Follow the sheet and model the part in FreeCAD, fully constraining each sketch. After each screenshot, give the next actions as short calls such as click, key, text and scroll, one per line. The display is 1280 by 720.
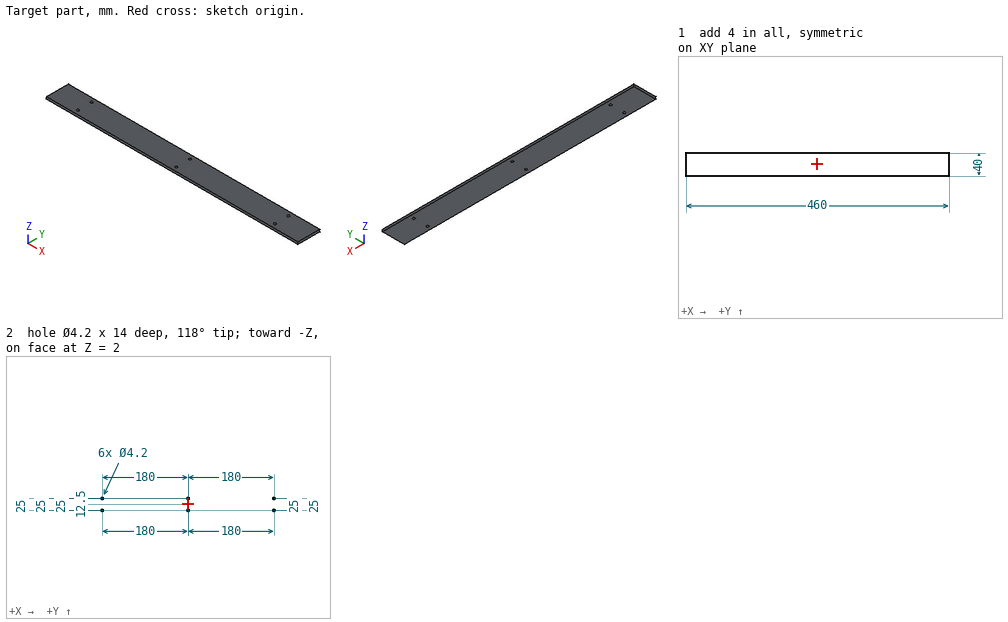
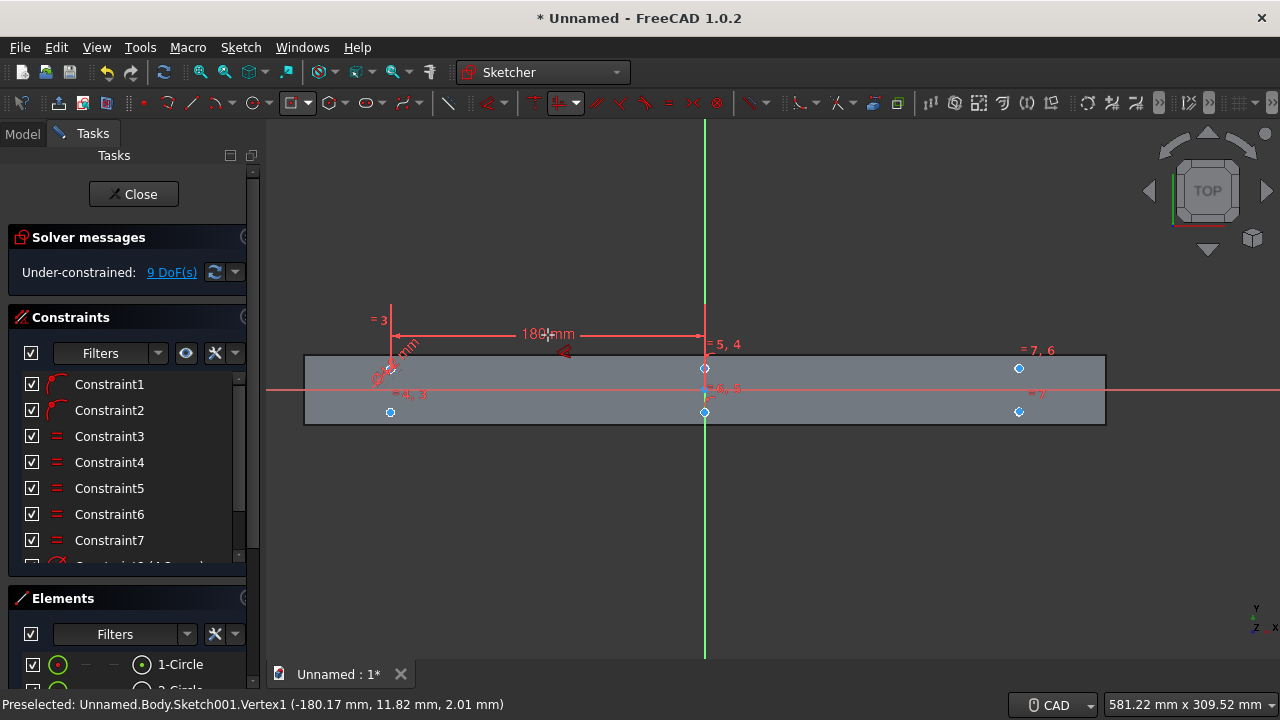
click(390, 413)
click(548, 447)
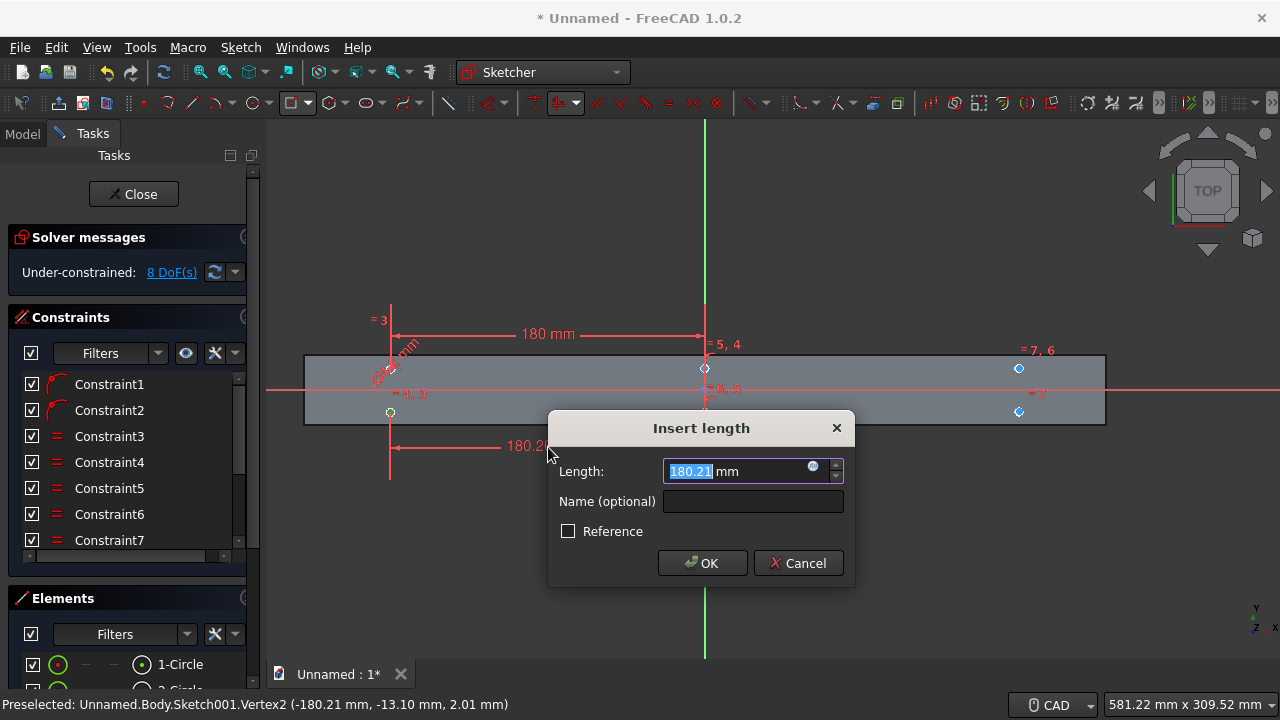
text(180)
key(Return)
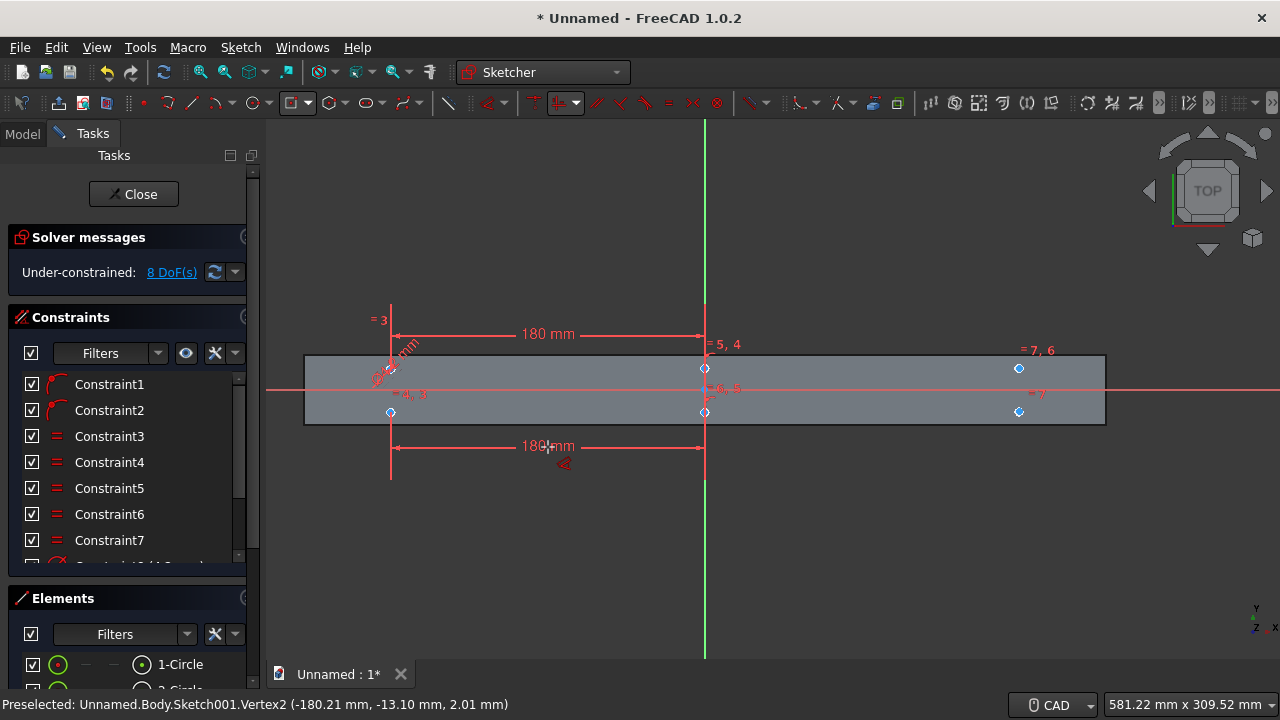
click(1019, 369)
click(862, 335)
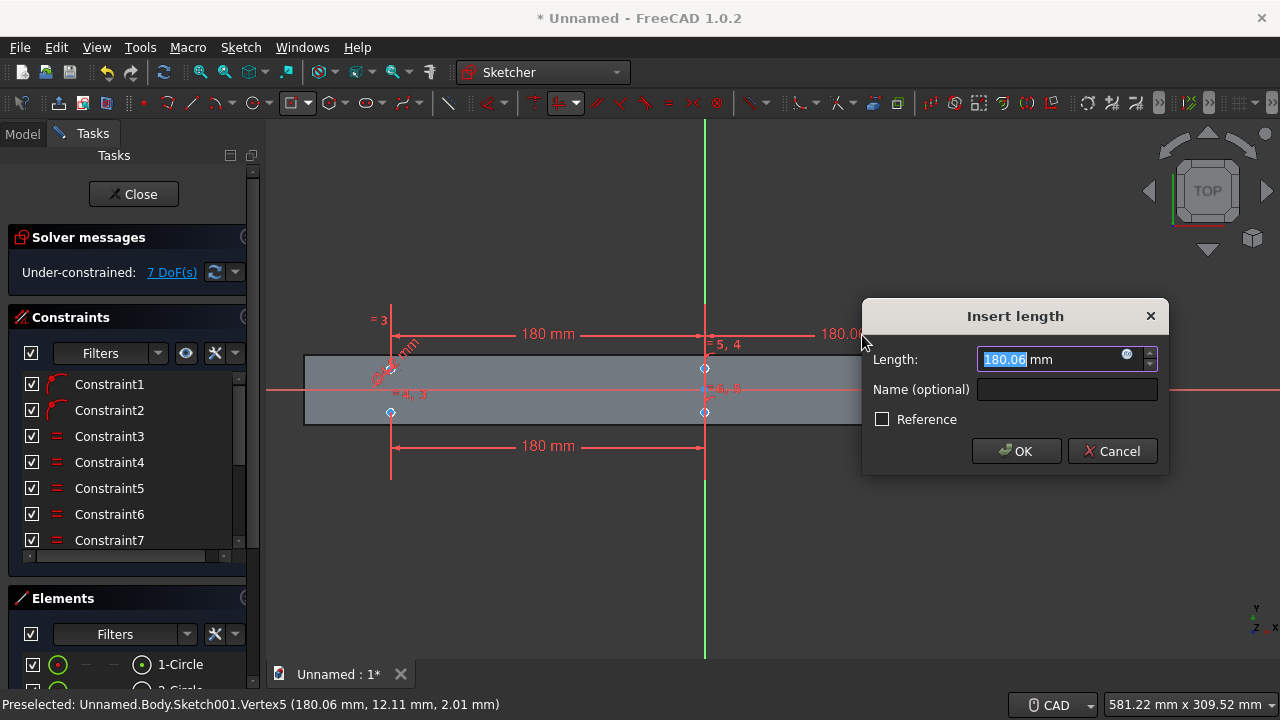
text(180)
key(Return)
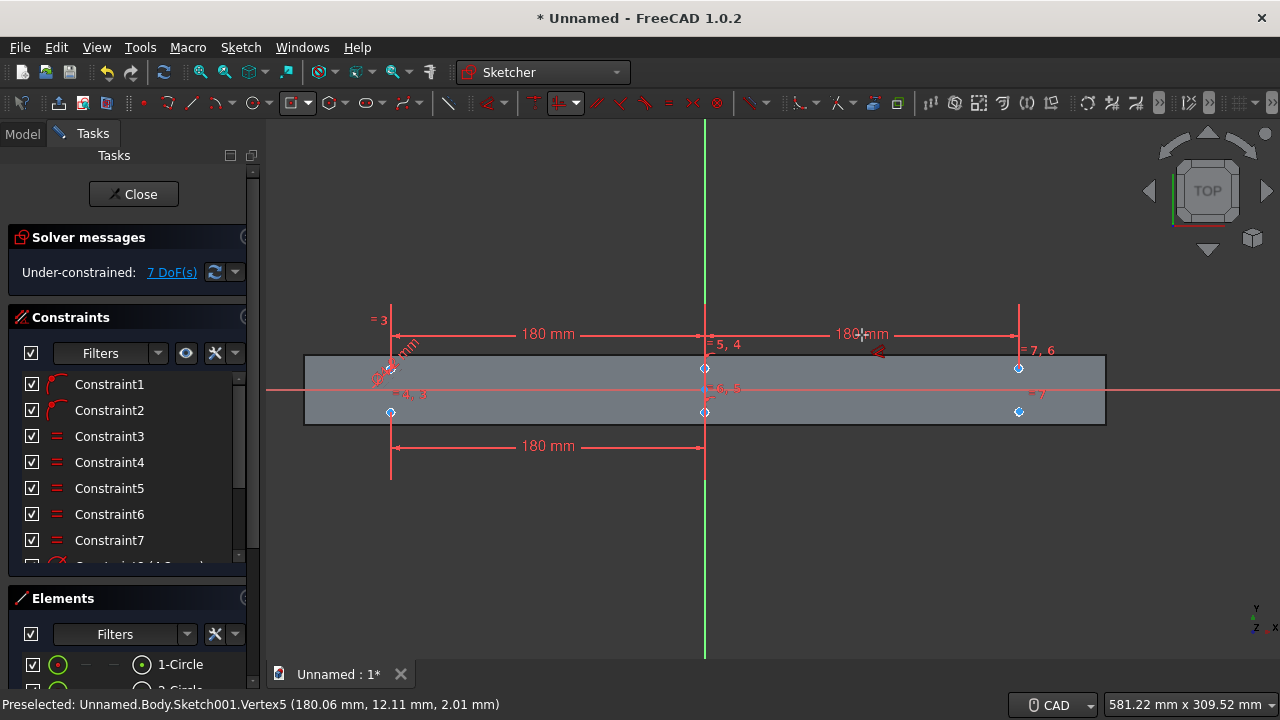
click(1019, 412)
click(862, 446)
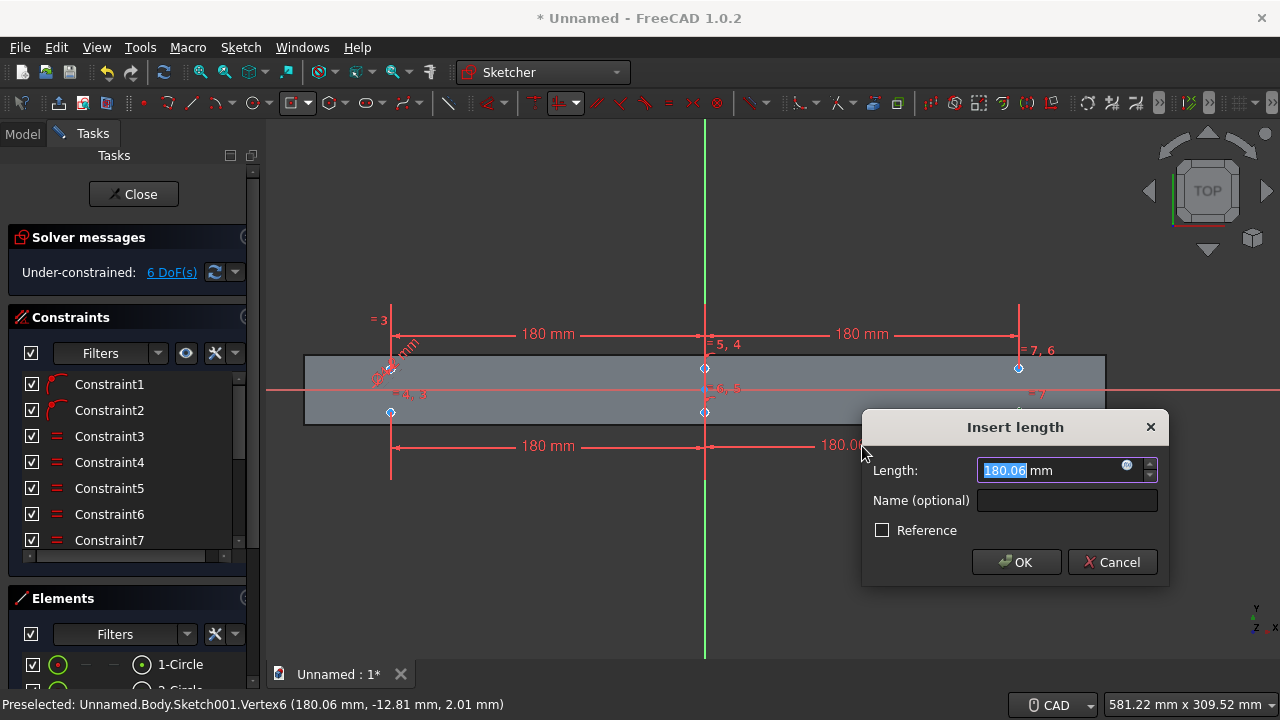
text(180)
key(Return)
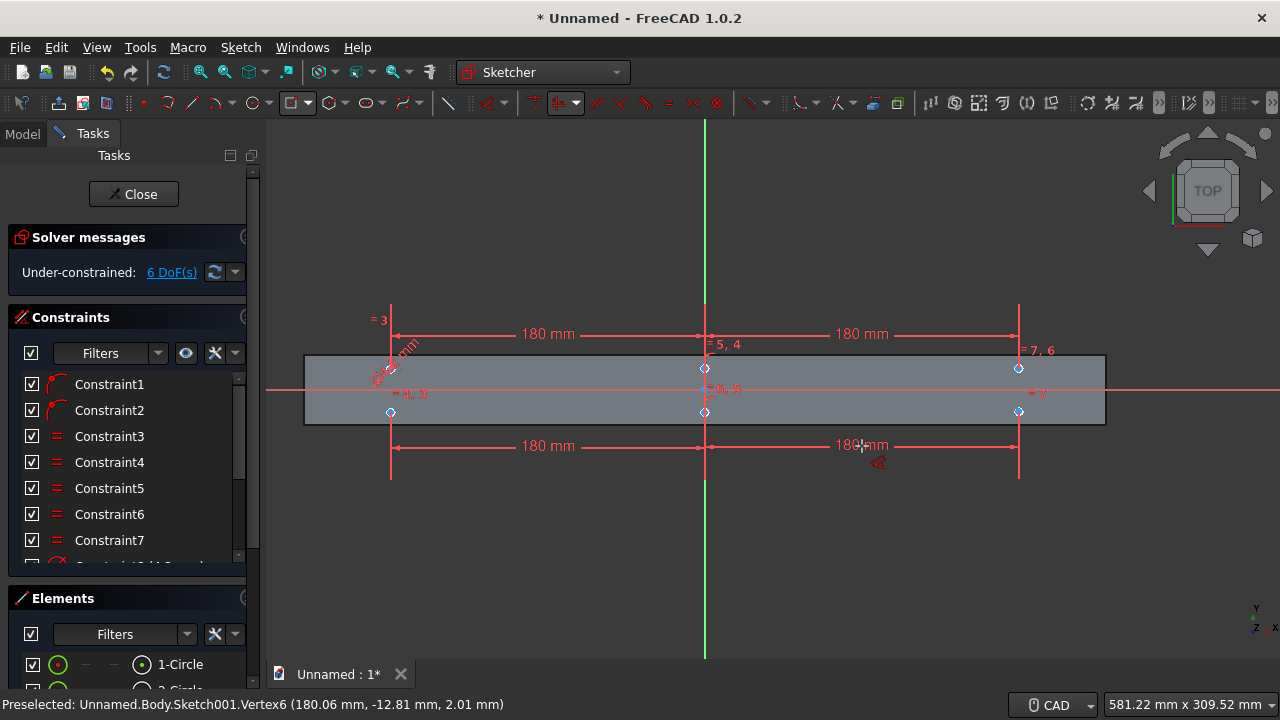
click(391, 369)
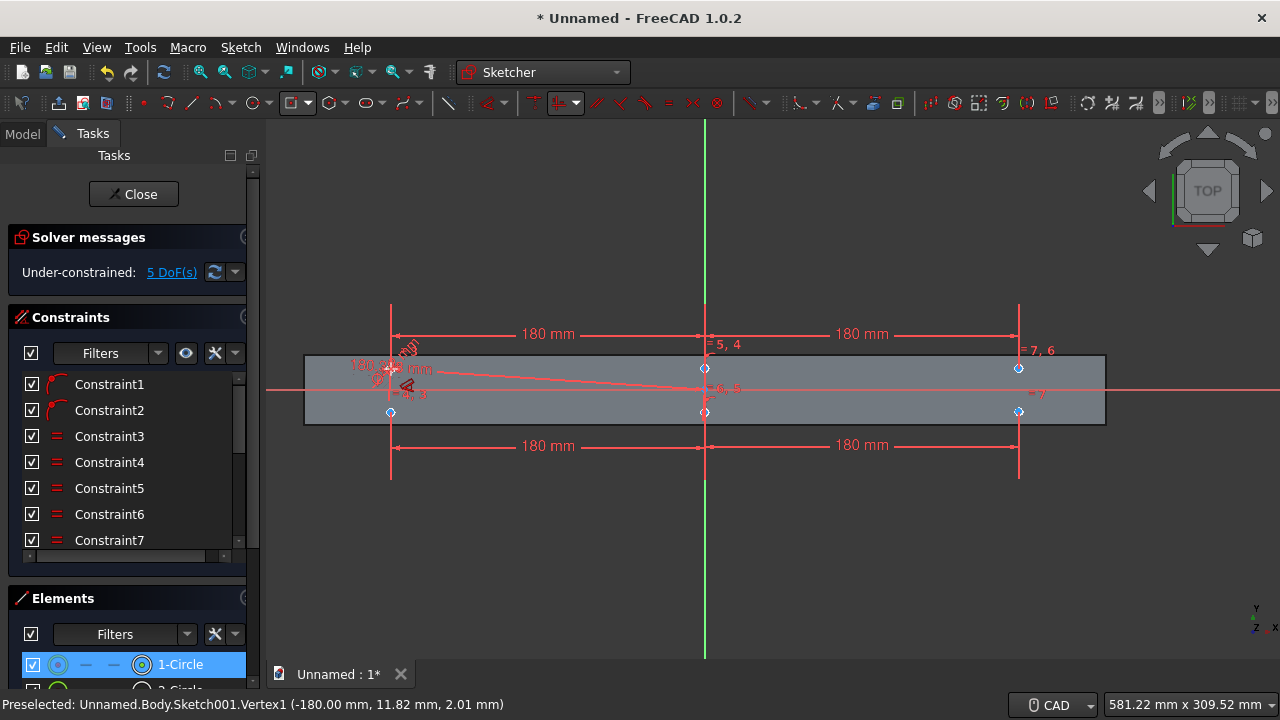
click(391, 413)
click(357, 406)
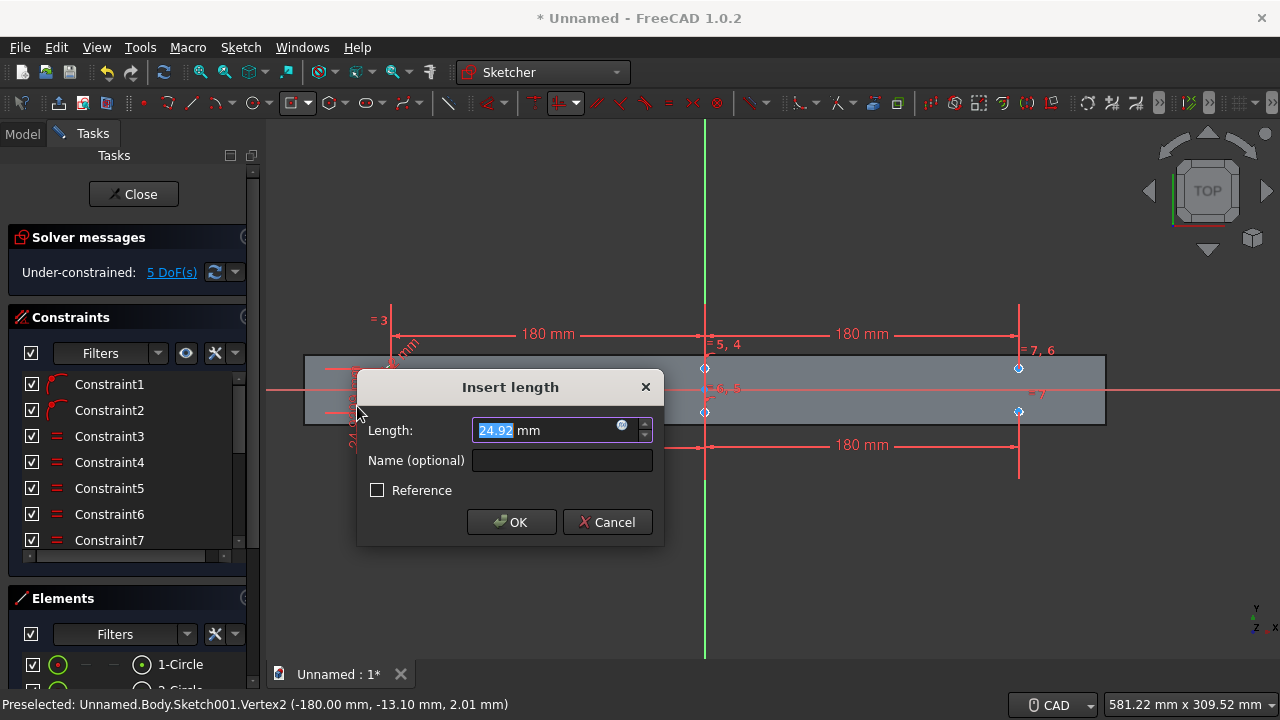
text(25)
key(Return)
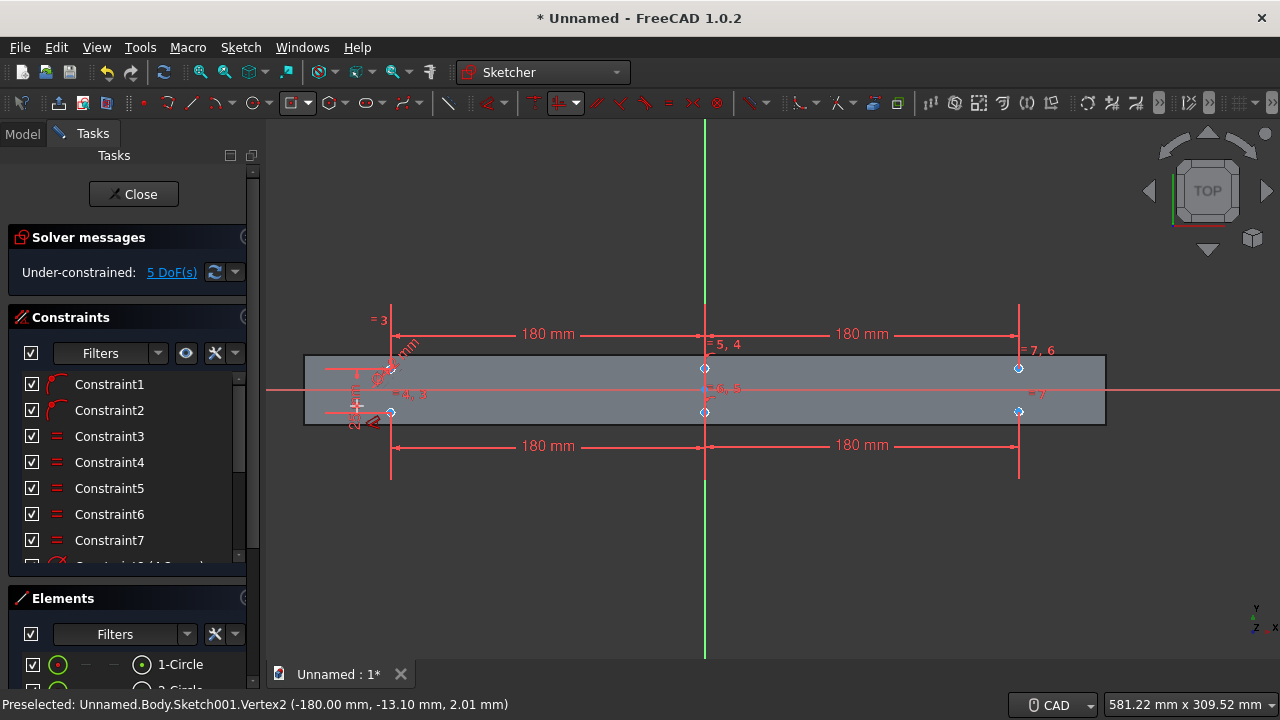
click(391, 413)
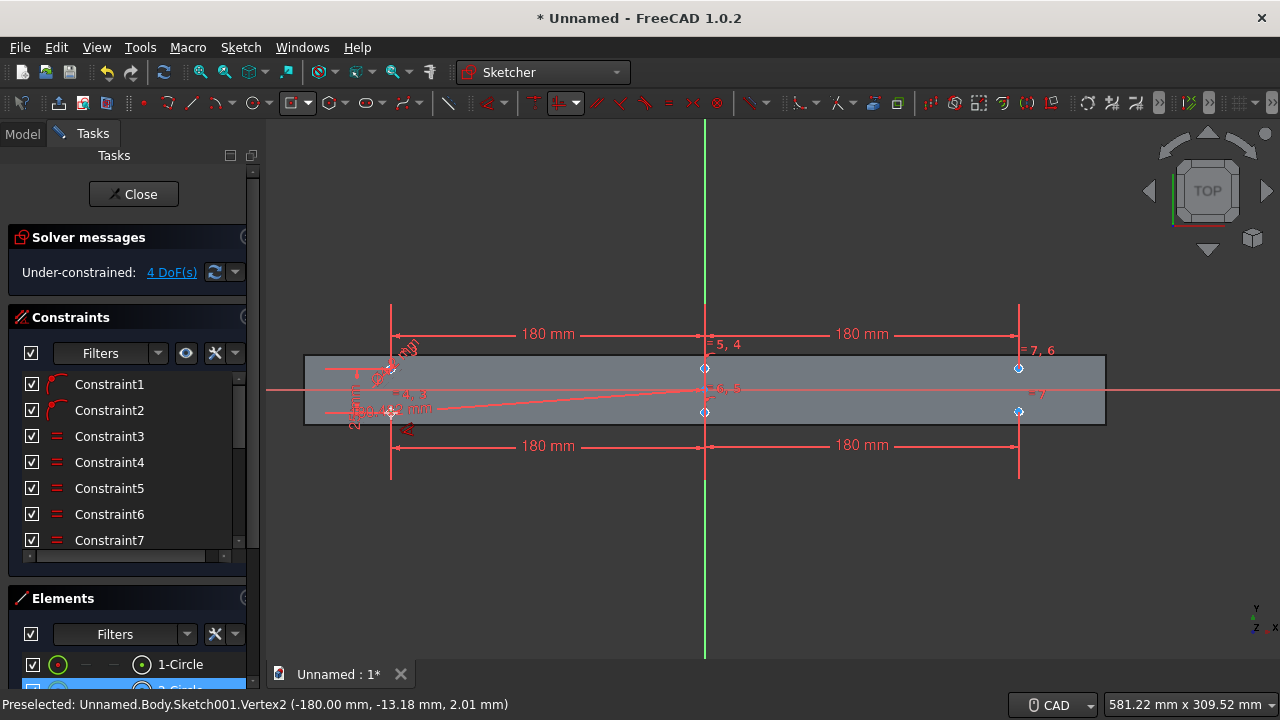
click(705, 369)
click(739, 375)